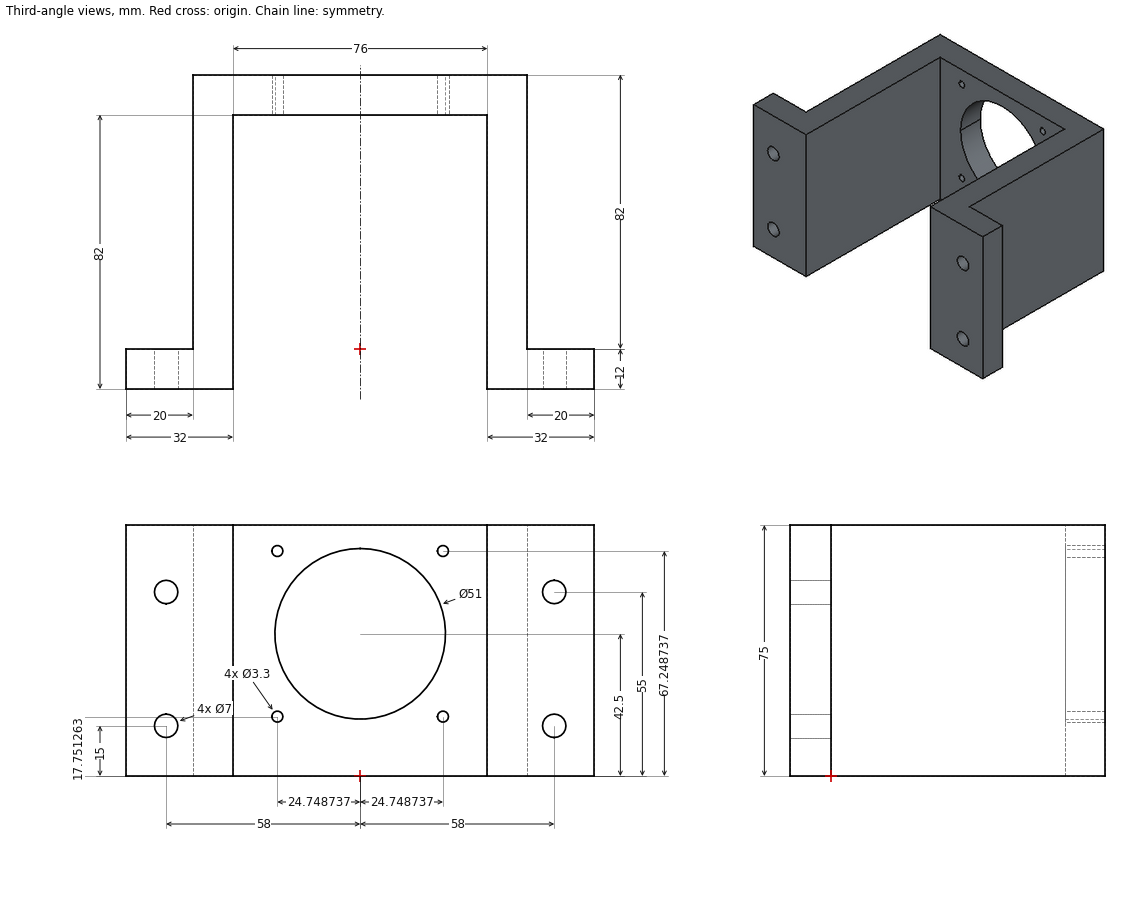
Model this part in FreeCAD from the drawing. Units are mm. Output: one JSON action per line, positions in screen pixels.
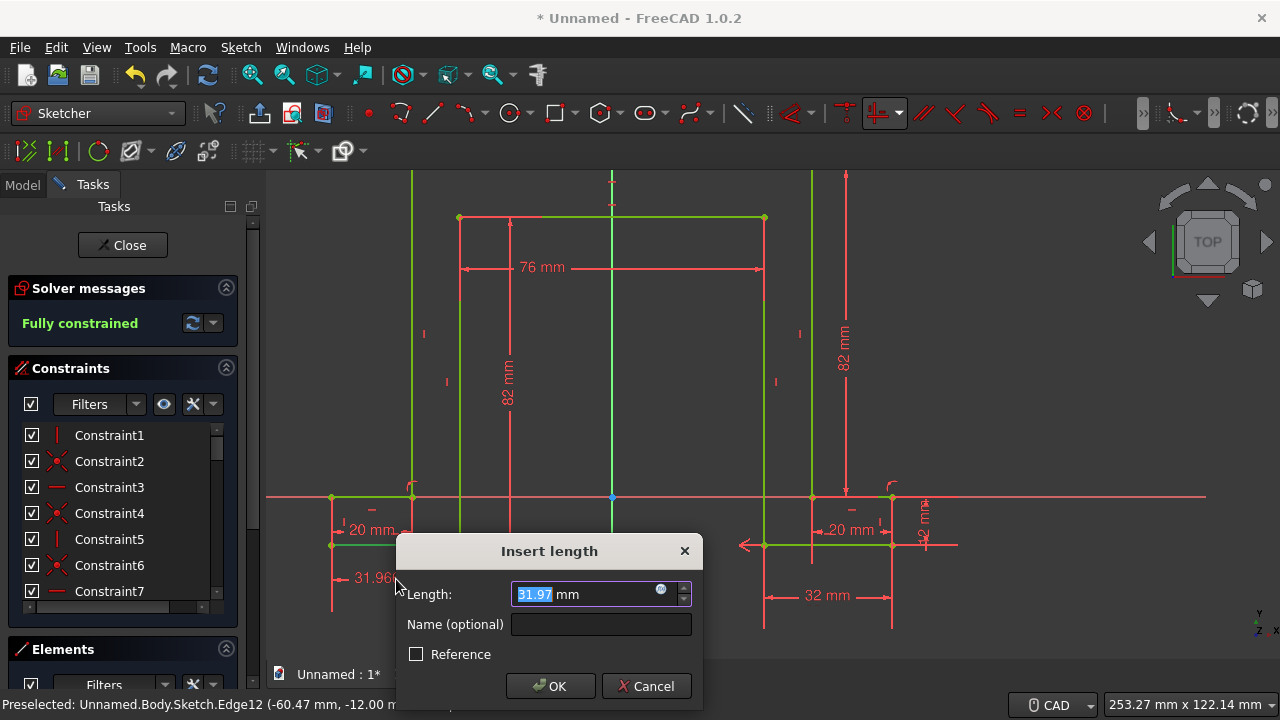
{"action": "type", "text": "32"}
{"action": "key", "text": "Return"}
{"action": "key", "text": "Escape"}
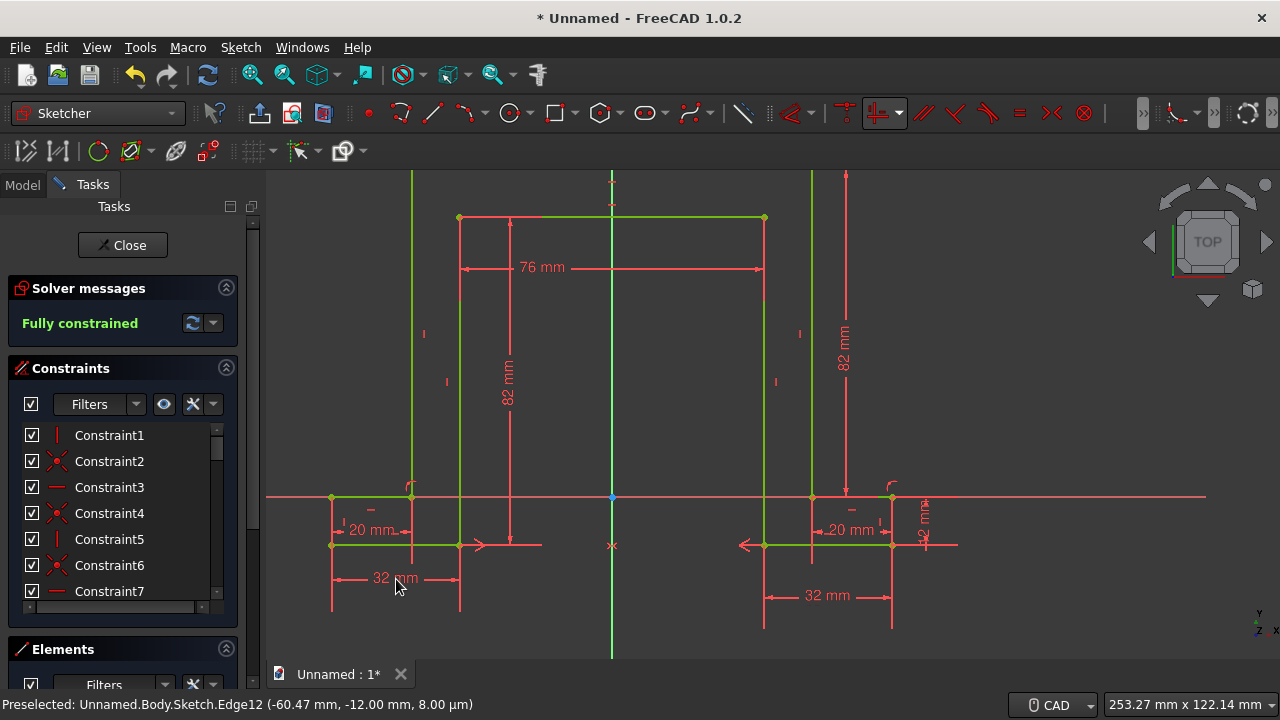
{"action": "left_click", "coordinate": [123, 245]}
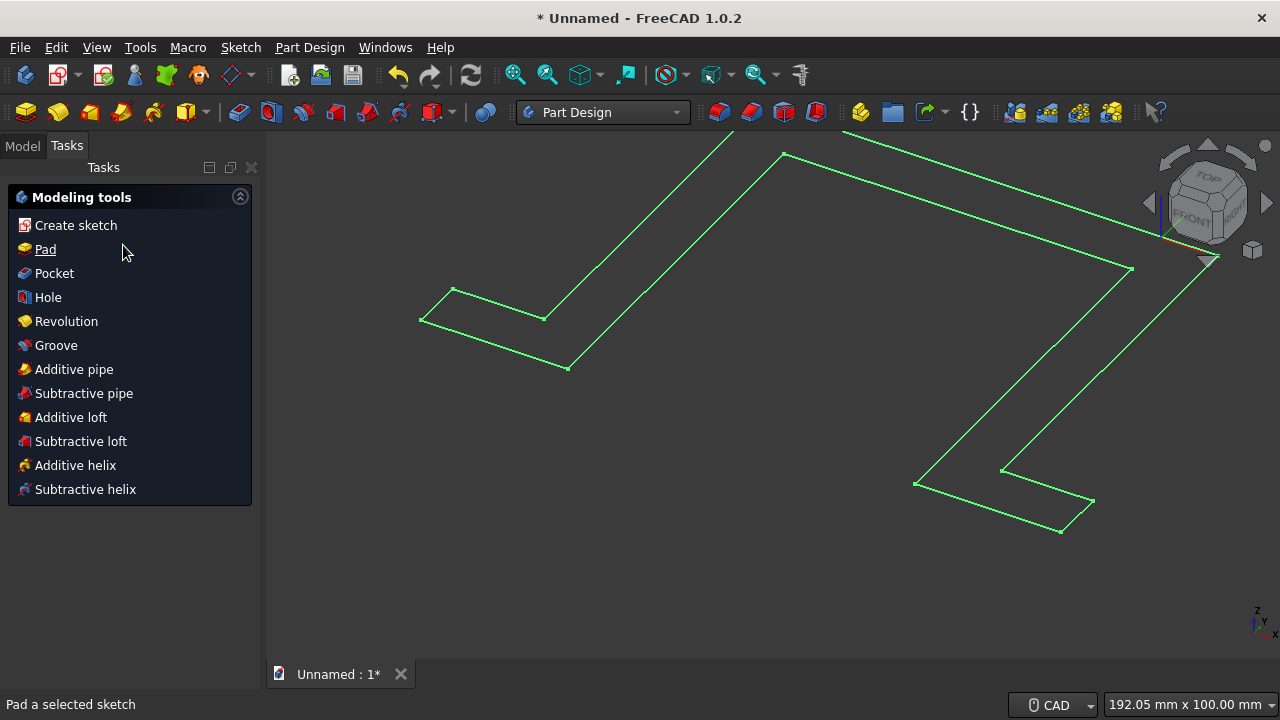
{"action": "left_click", "coordinate": [26, 112]}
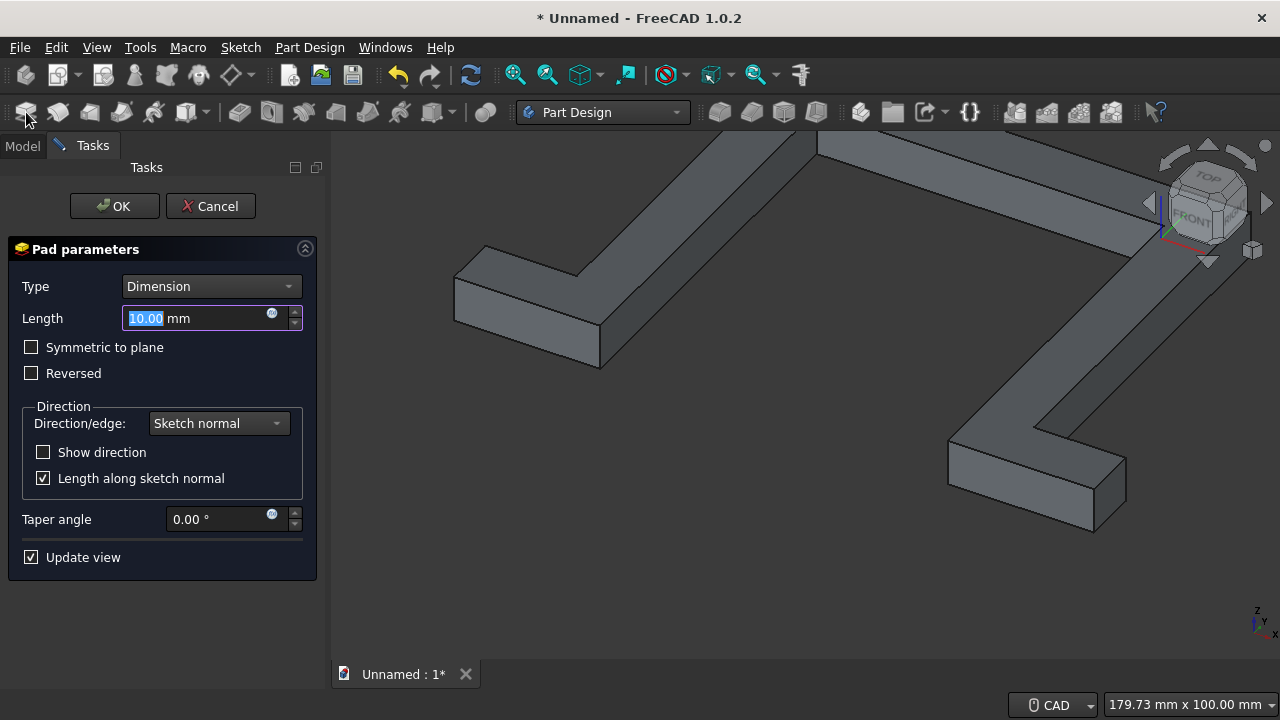
{"action": "type", "text": "75"}
{"action": "key", "text": "Tab"}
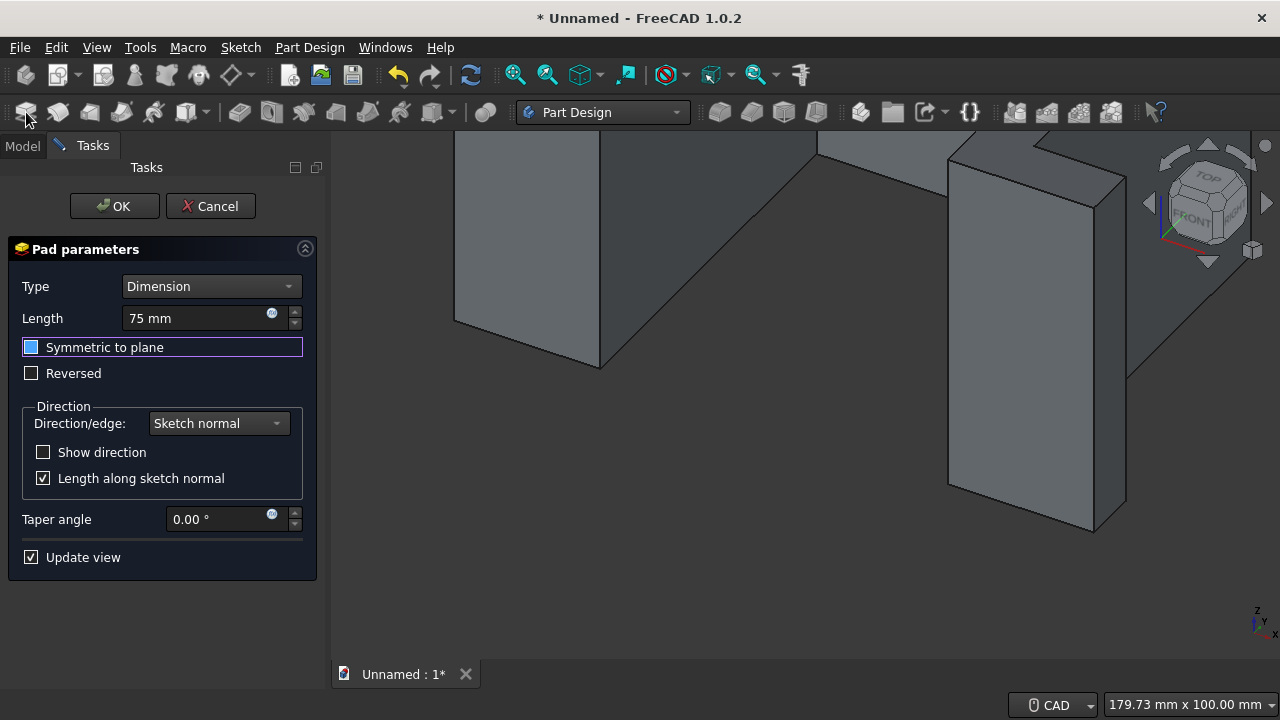
{"action": "left_click", "coordinate": [115, 206]}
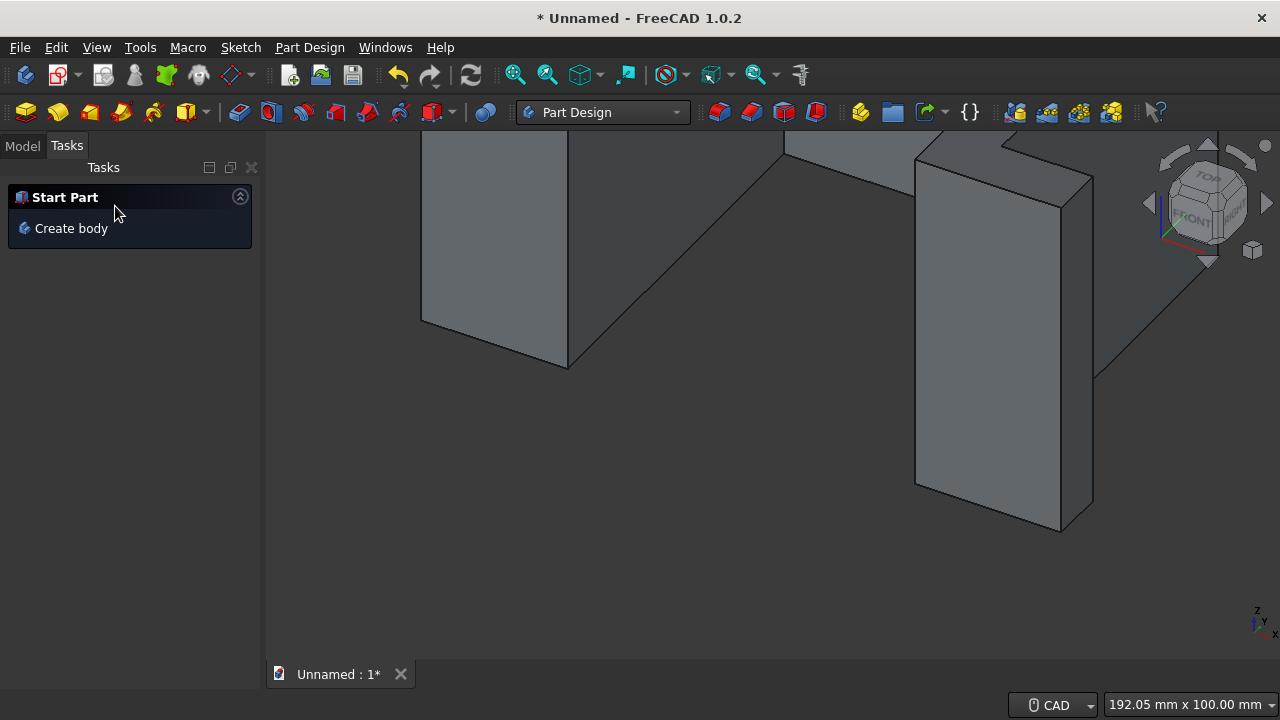
{"action": "left_click", "coordinate": [516, 76]}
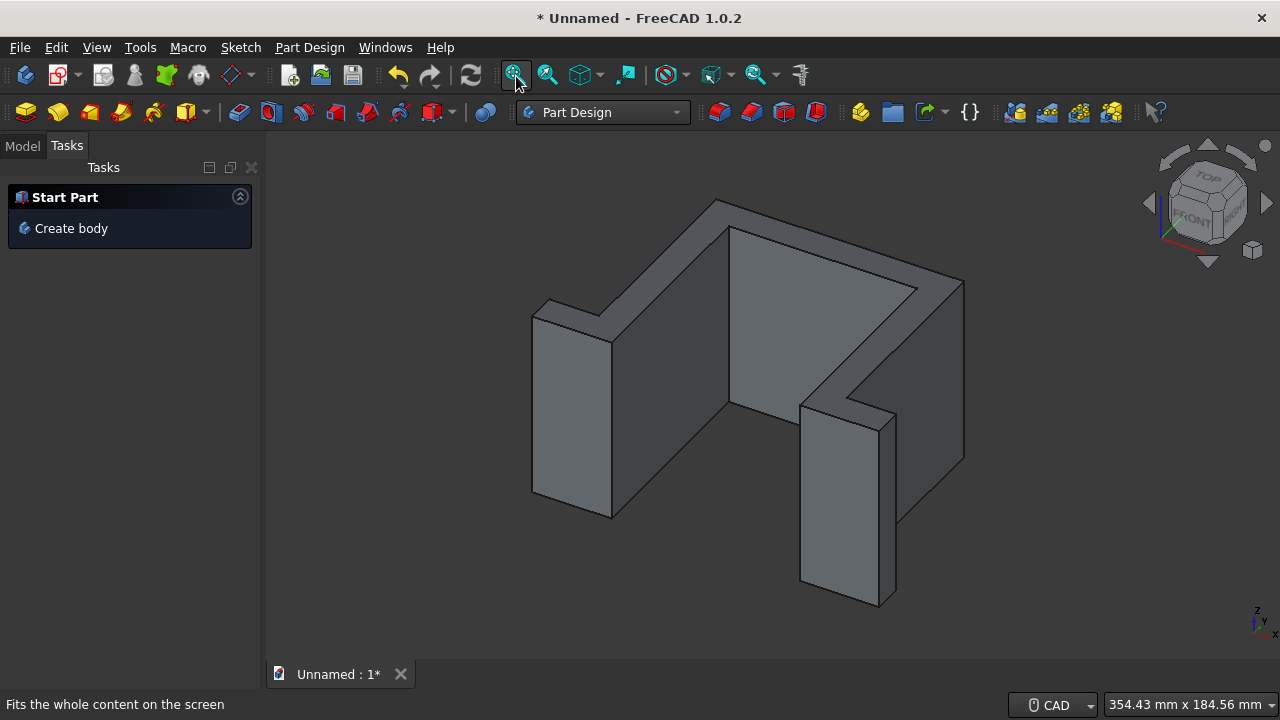
{"action": "key", "text": "4"}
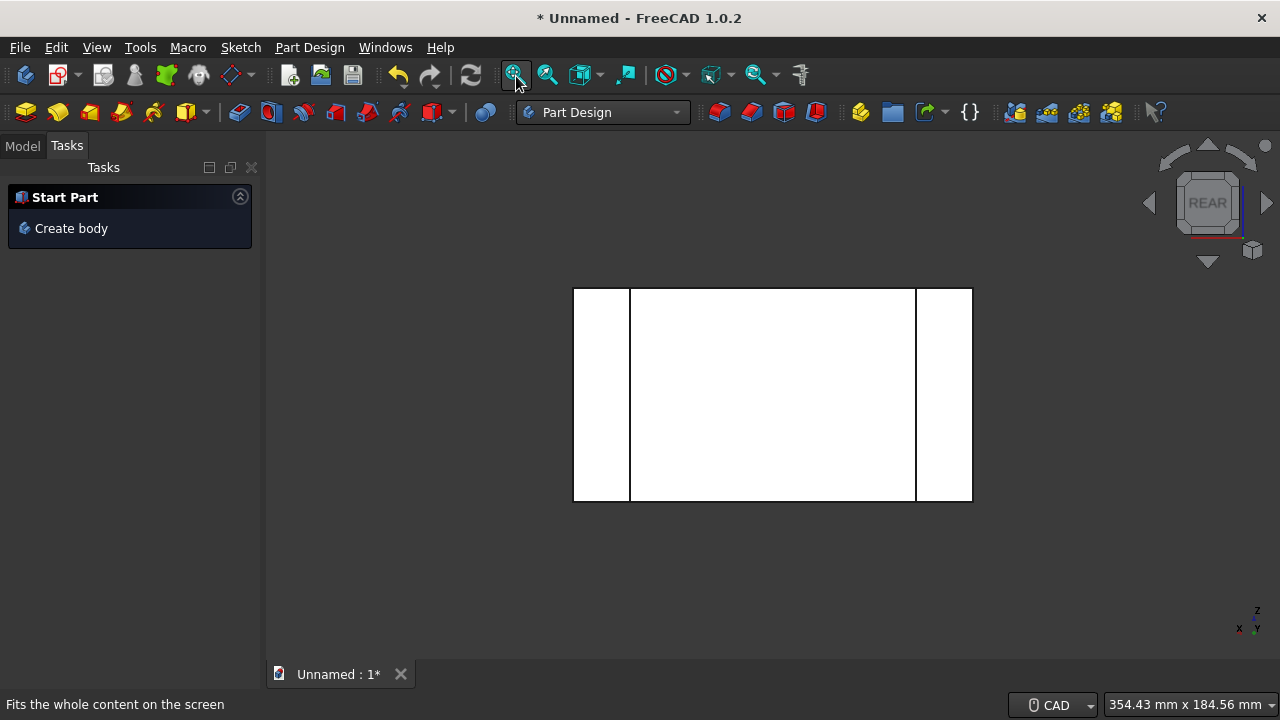
{"action": "left_click", "coordinate": [516, 76]}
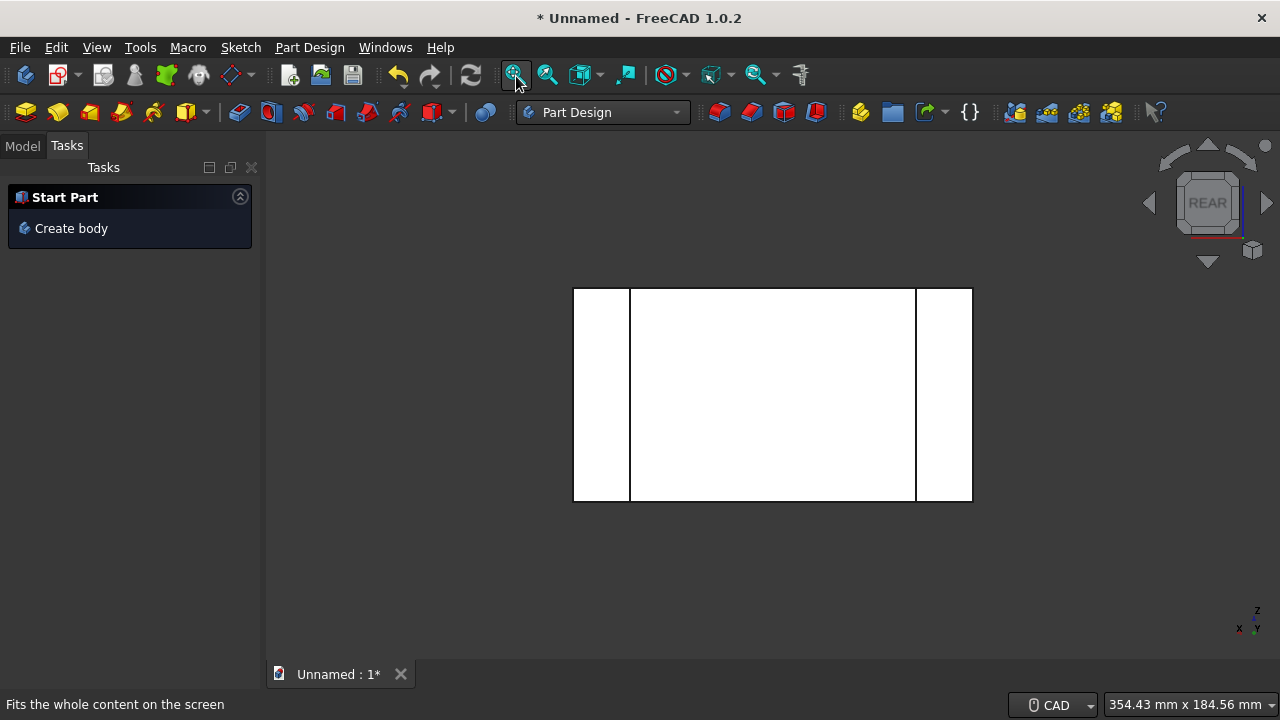
{"action": "left_click", "coordinate": [773, 394]}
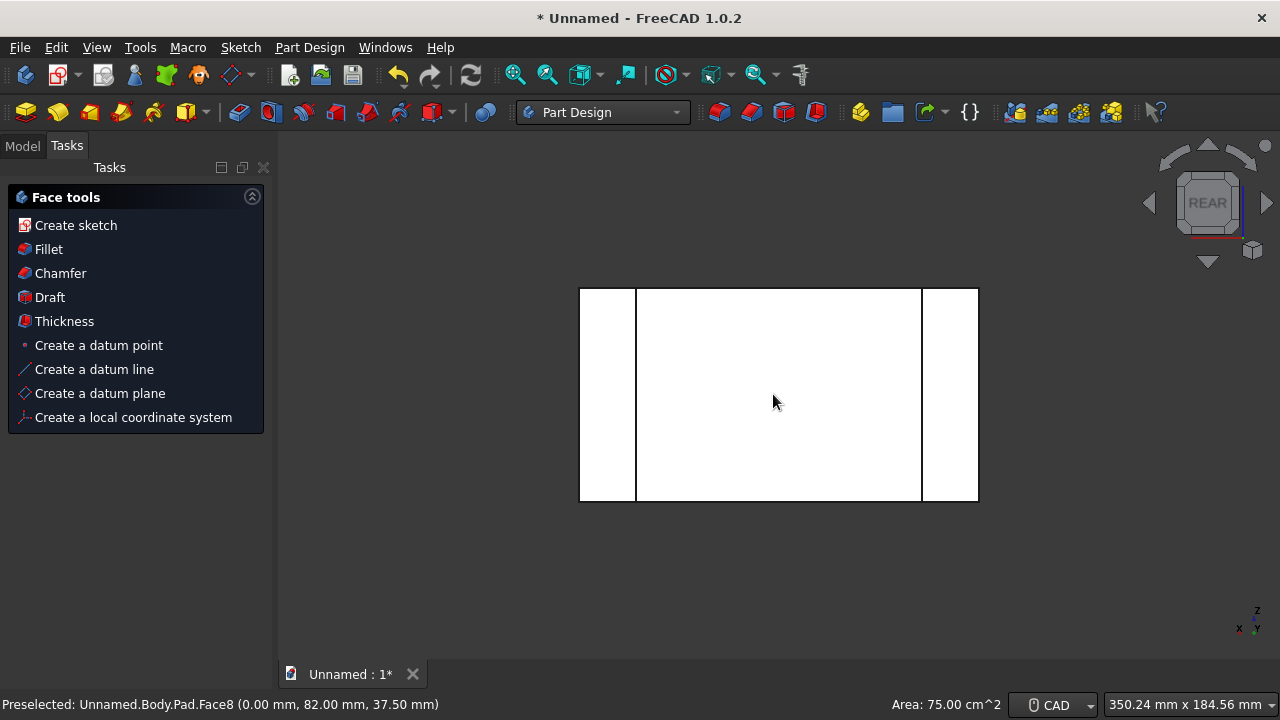
{"action": "left_click", "coordinate": [58, 76]}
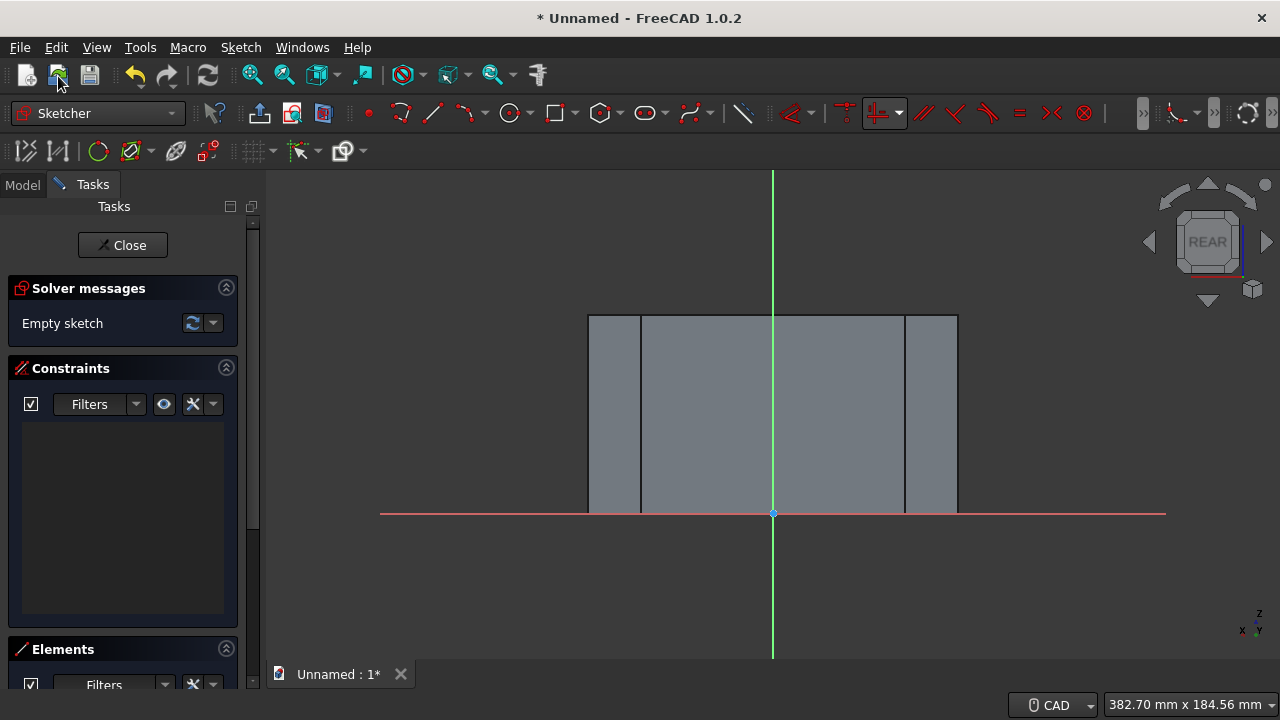
{"action": "scroll", "coordinate": [856, 435], "scroll_direction": "up", "scroll_amount": 3}